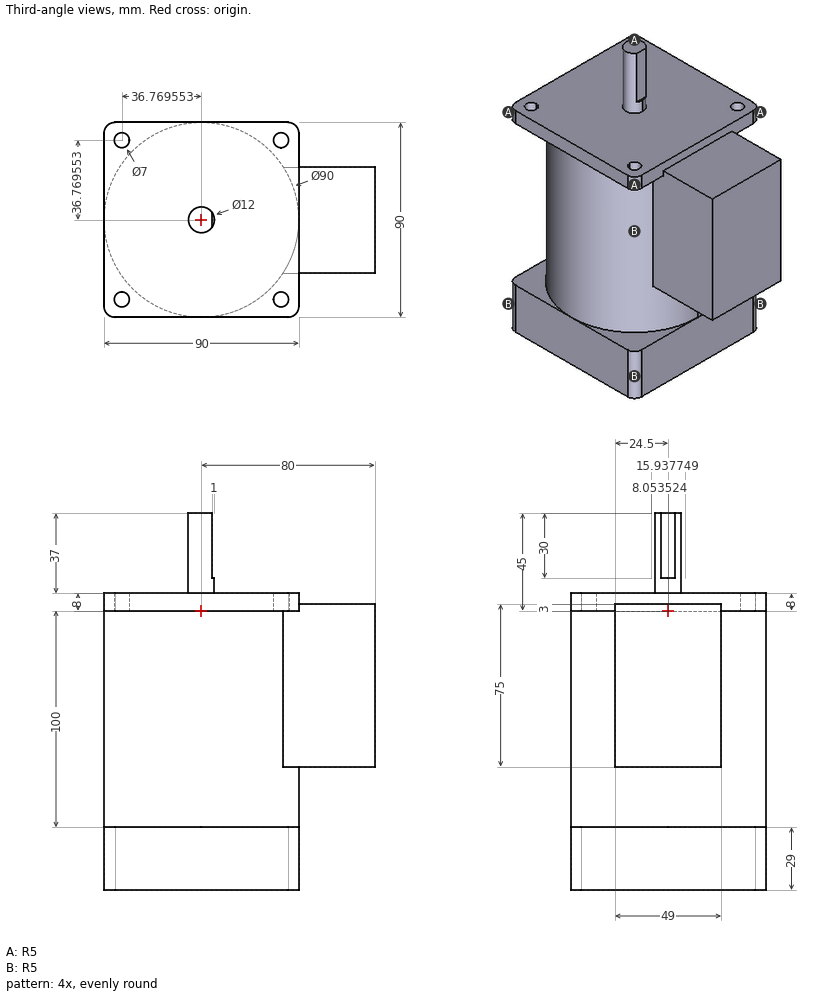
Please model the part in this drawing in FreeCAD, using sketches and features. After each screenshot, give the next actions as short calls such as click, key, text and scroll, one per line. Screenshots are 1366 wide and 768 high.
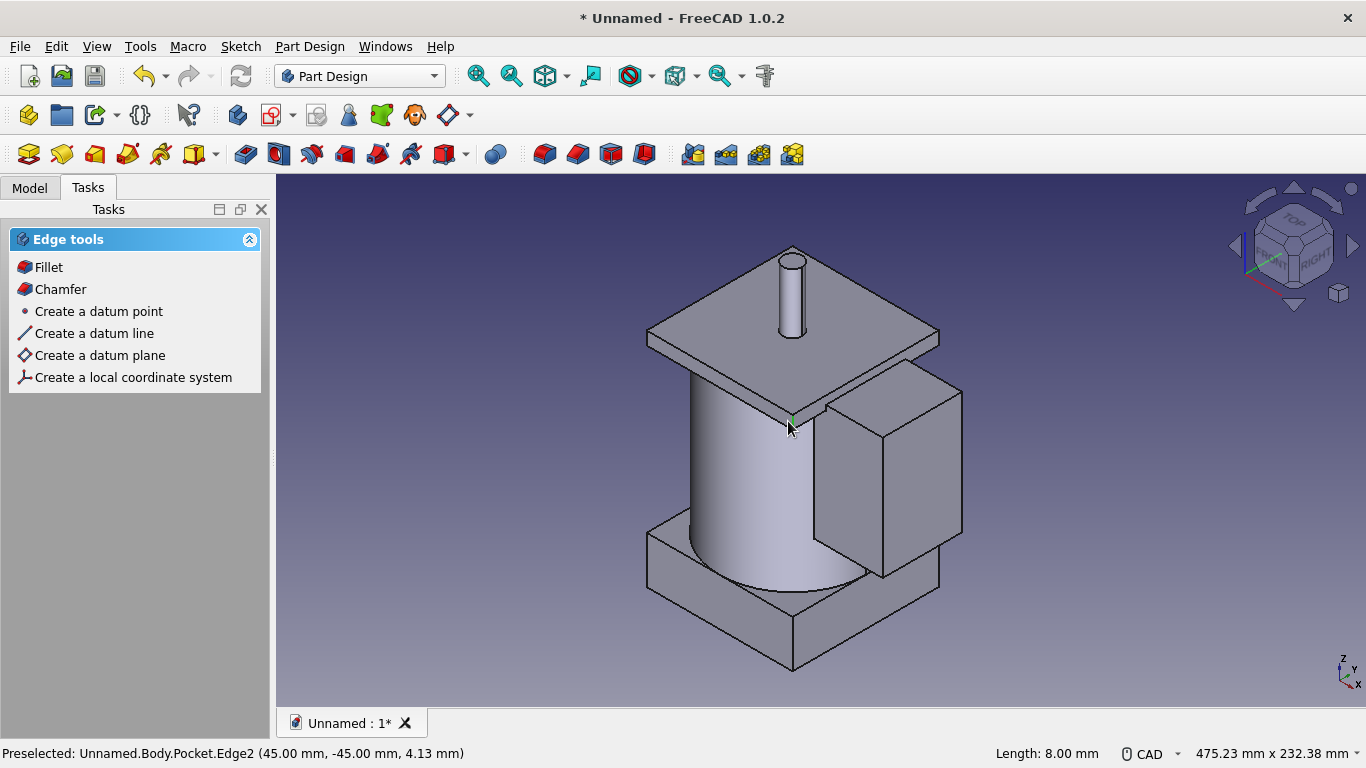
scroll(793, 253, up, 4)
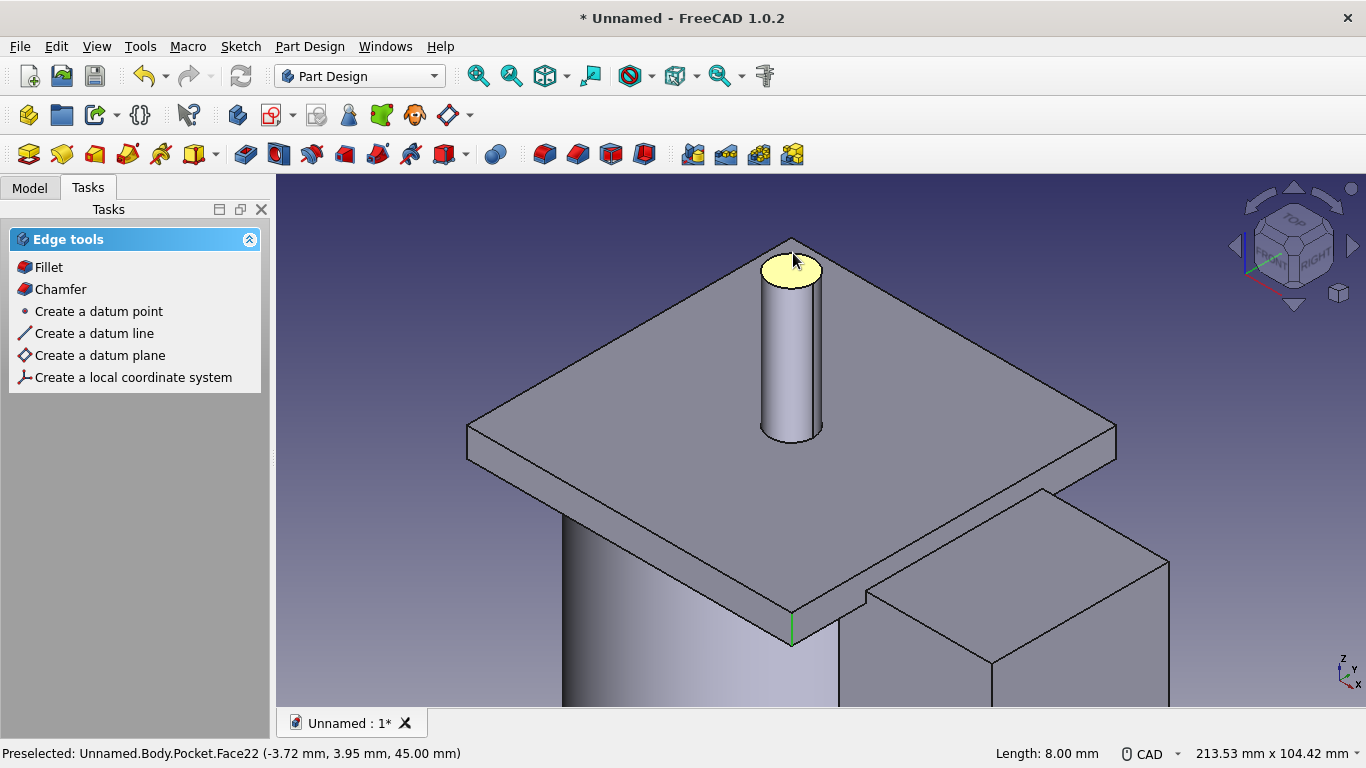
click(479, 76)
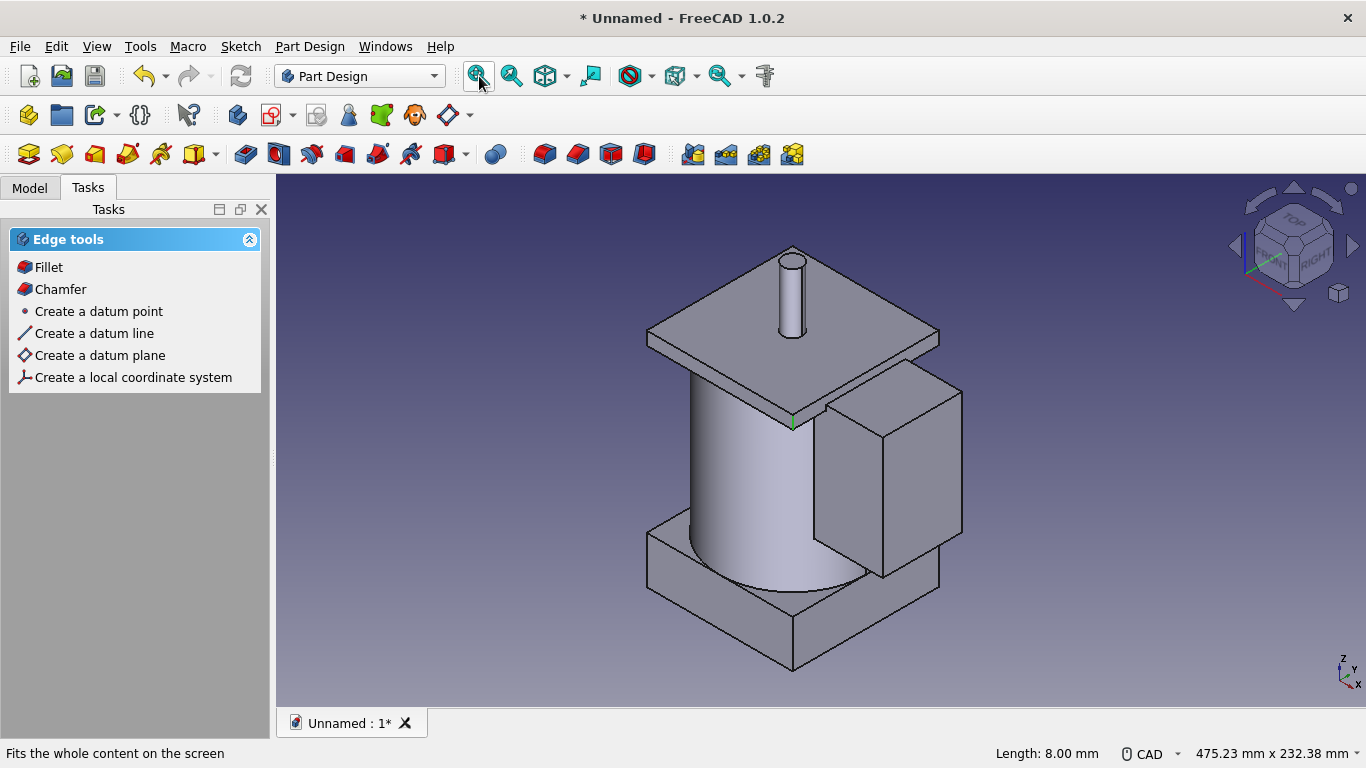
key(2)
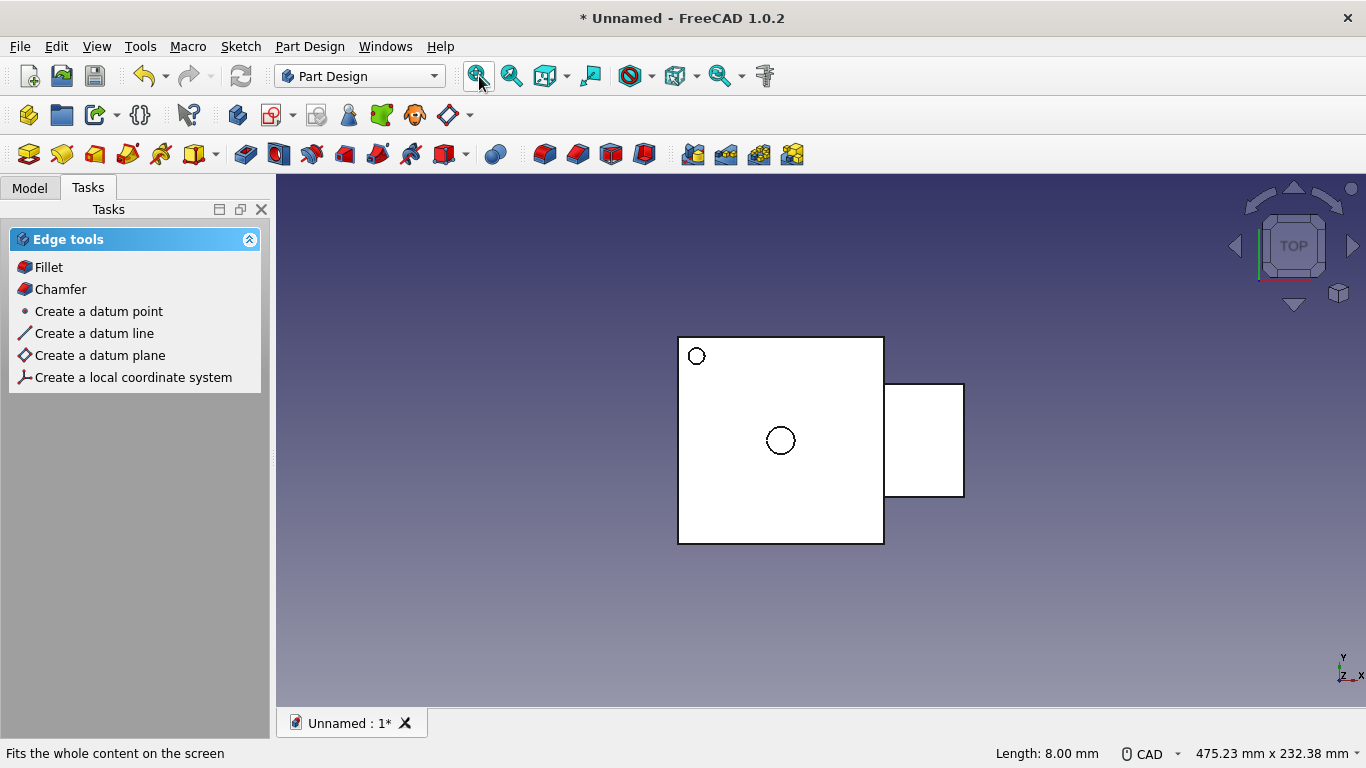
key(v)
key(f)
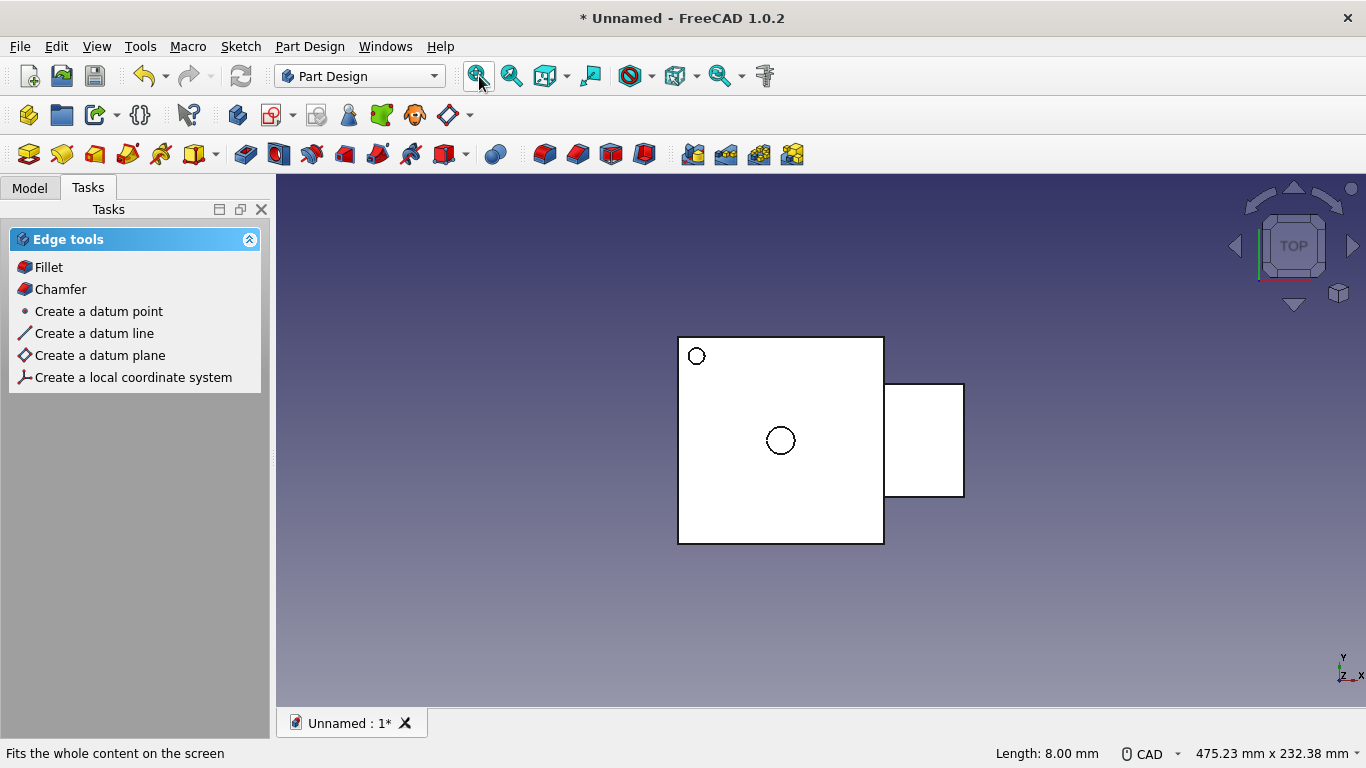
scroll(678, 336, up, 4)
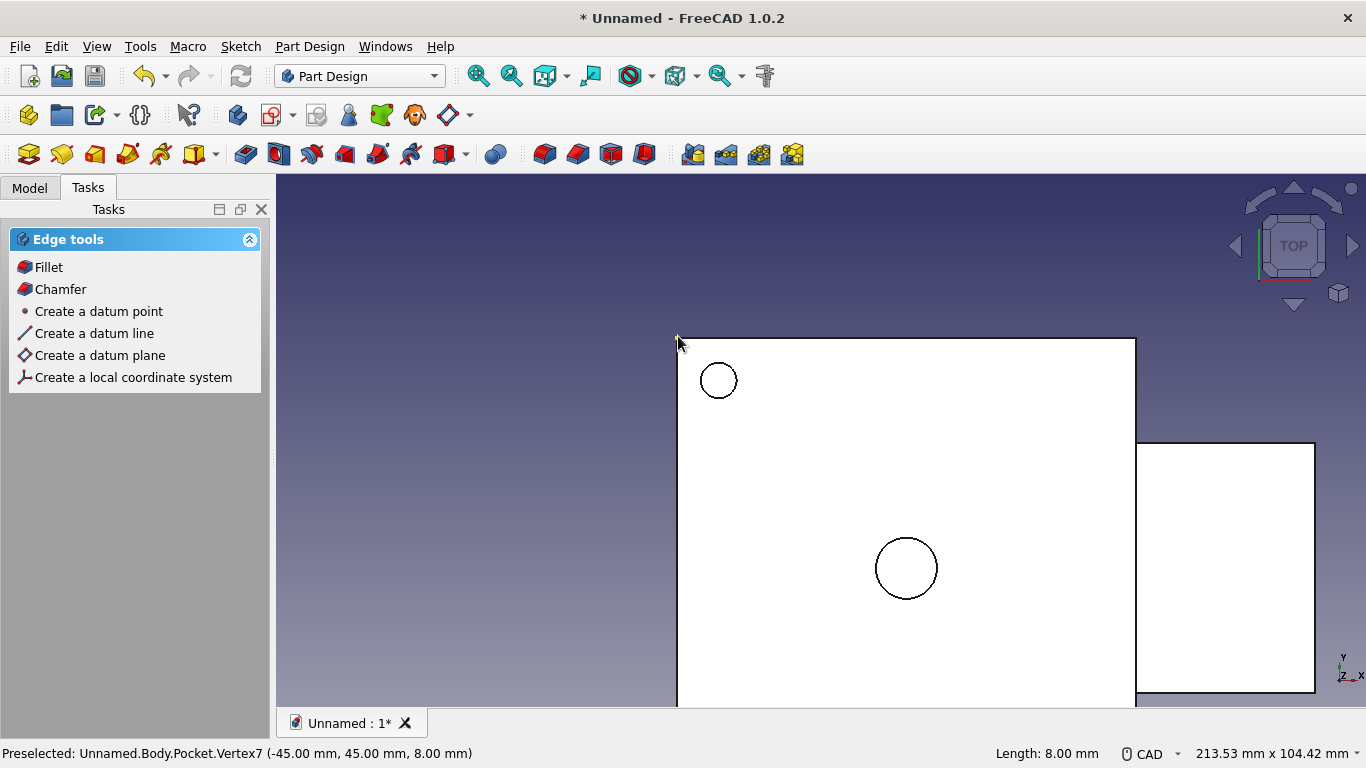
key(v)
key(f)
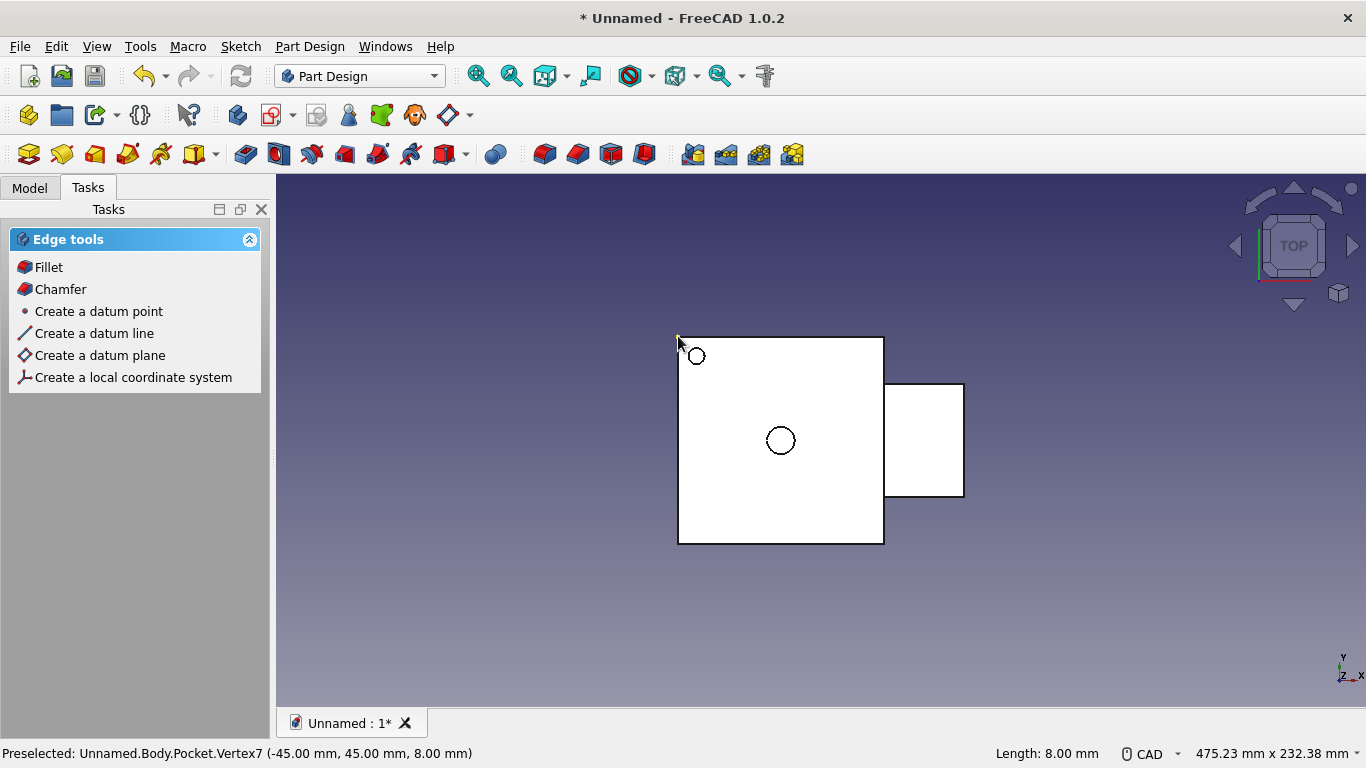
key(0)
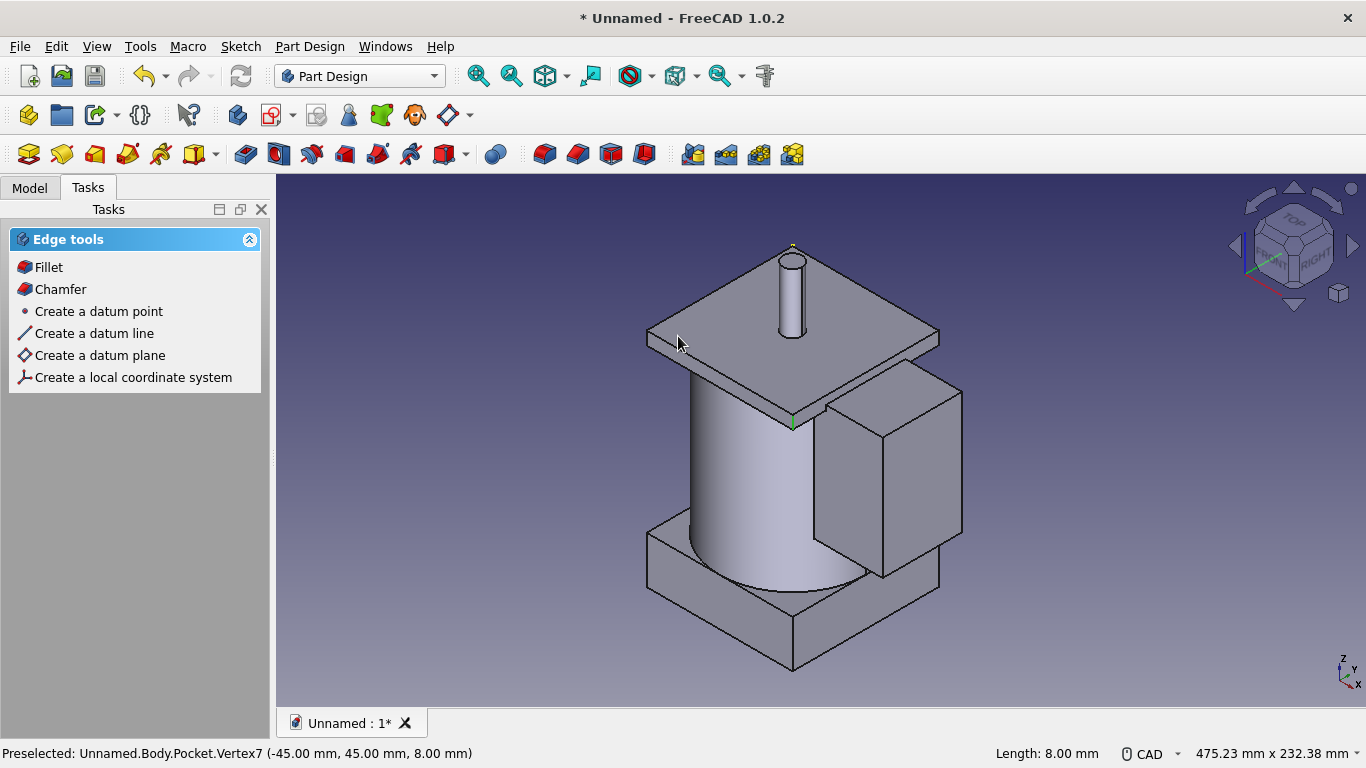
scroll(793, 253, up, 4)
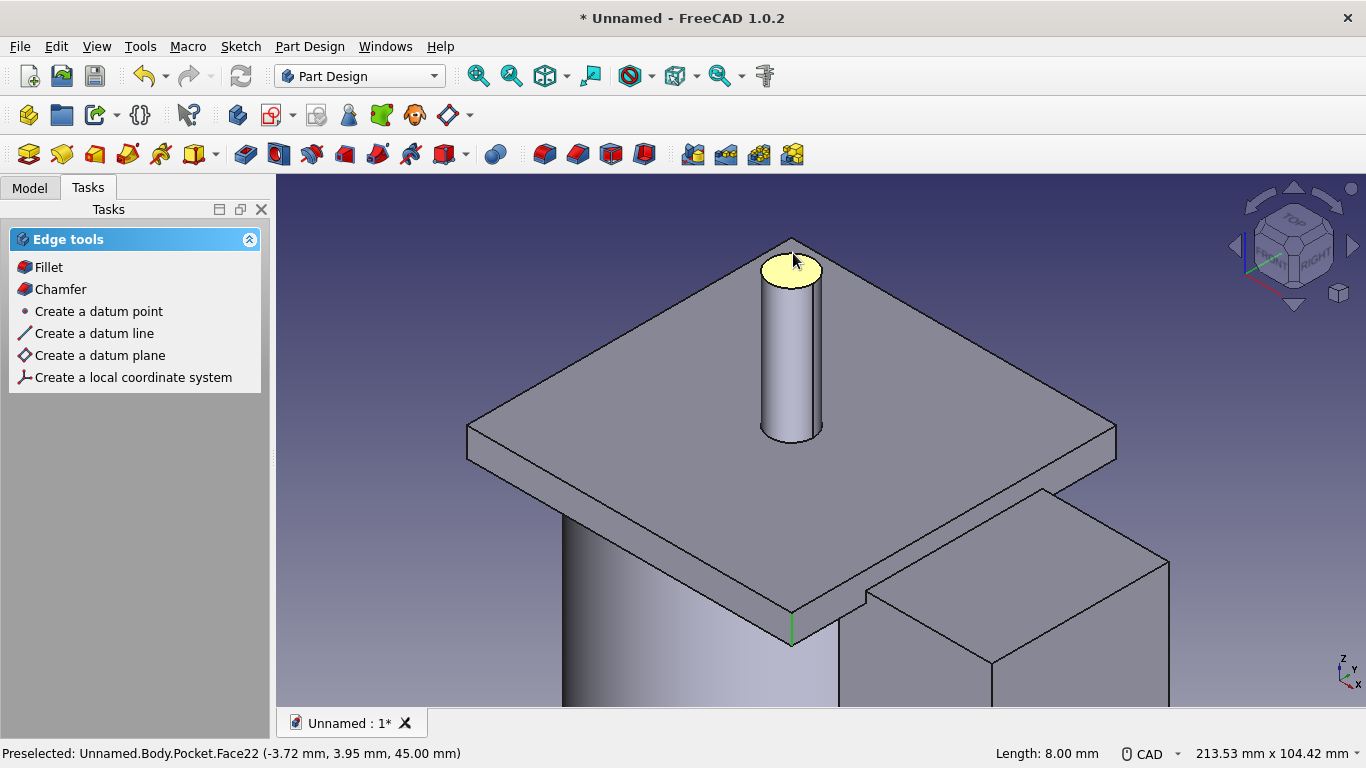
click(479, 76)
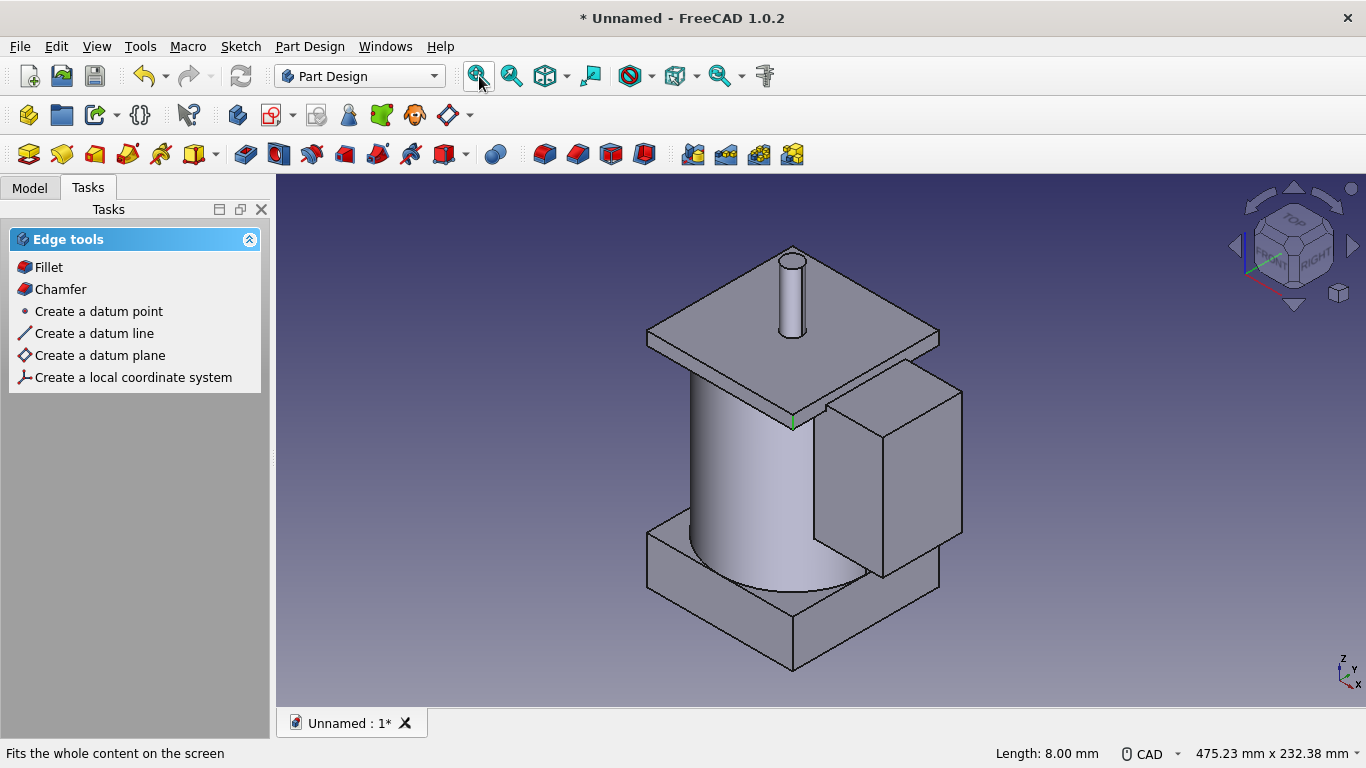
key(1)